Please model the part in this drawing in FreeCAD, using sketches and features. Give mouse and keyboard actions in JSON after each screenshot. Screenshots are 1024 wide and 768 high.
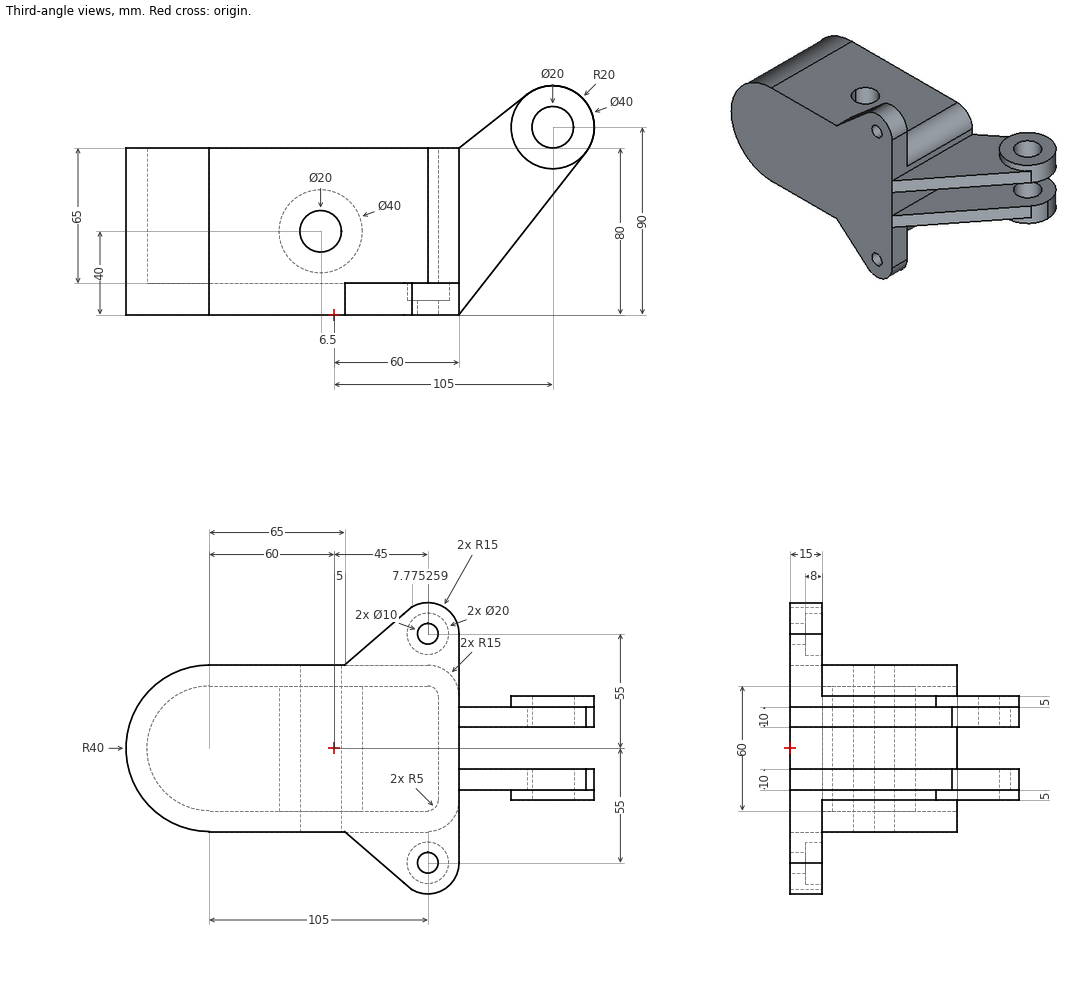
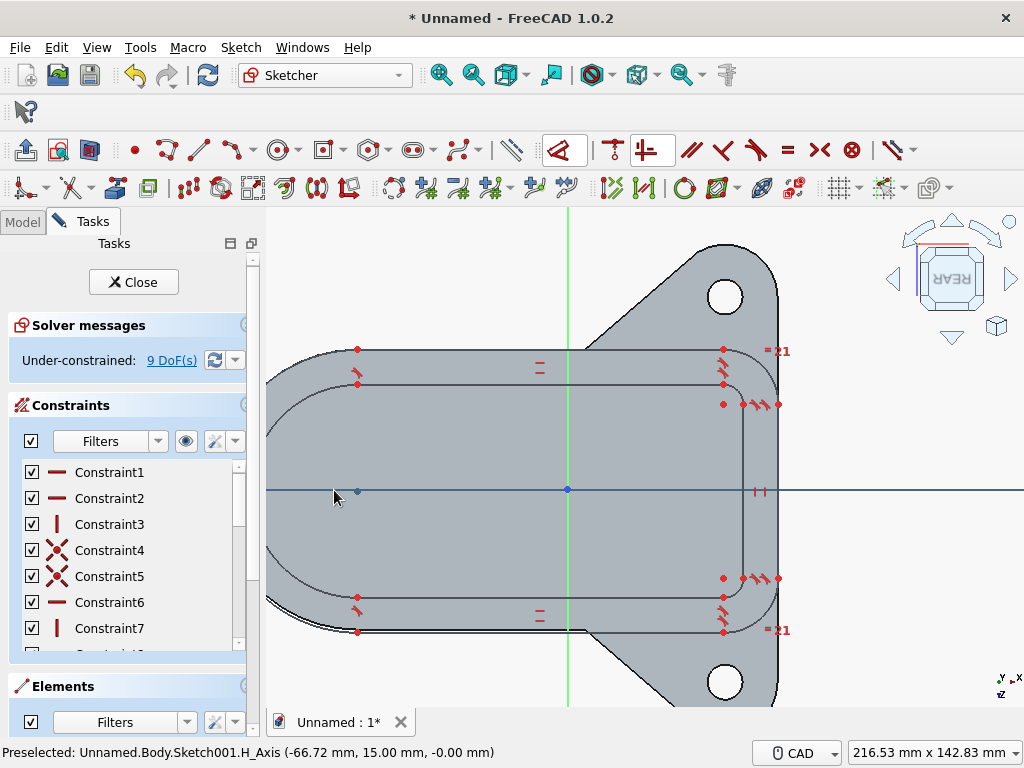
{"action": "left_click", "coordinate": [614, 150]}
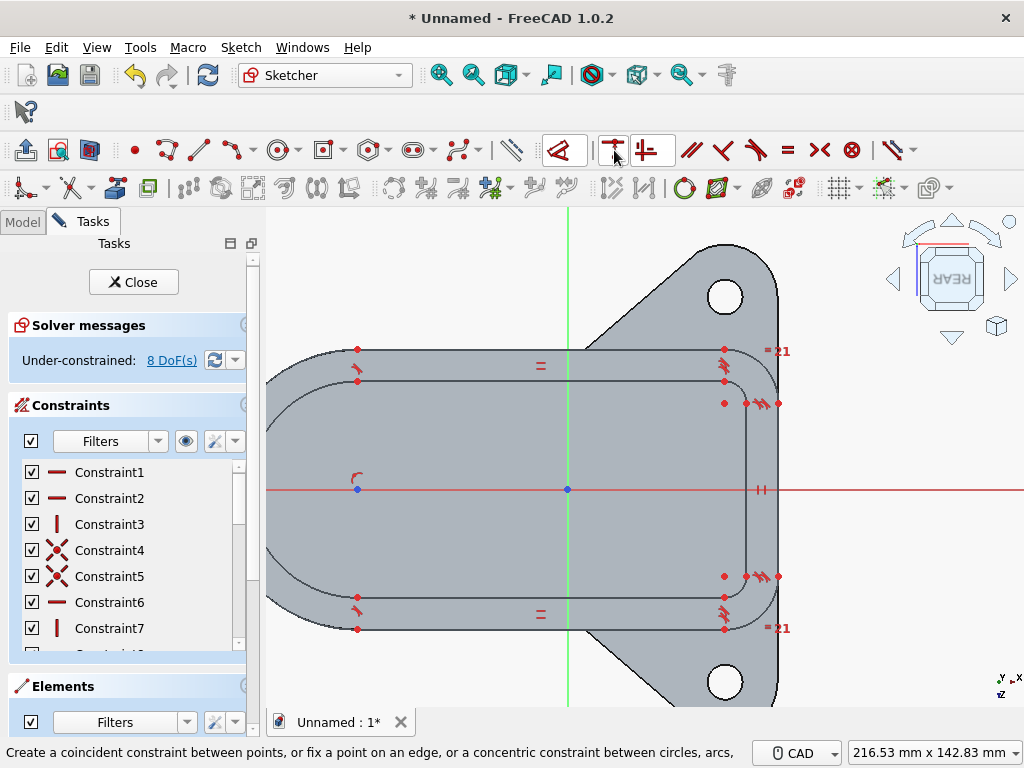
{"action": "scroll", "coordinate": [737, 391], "scroll_direction": "down", "scroll_amount": 2}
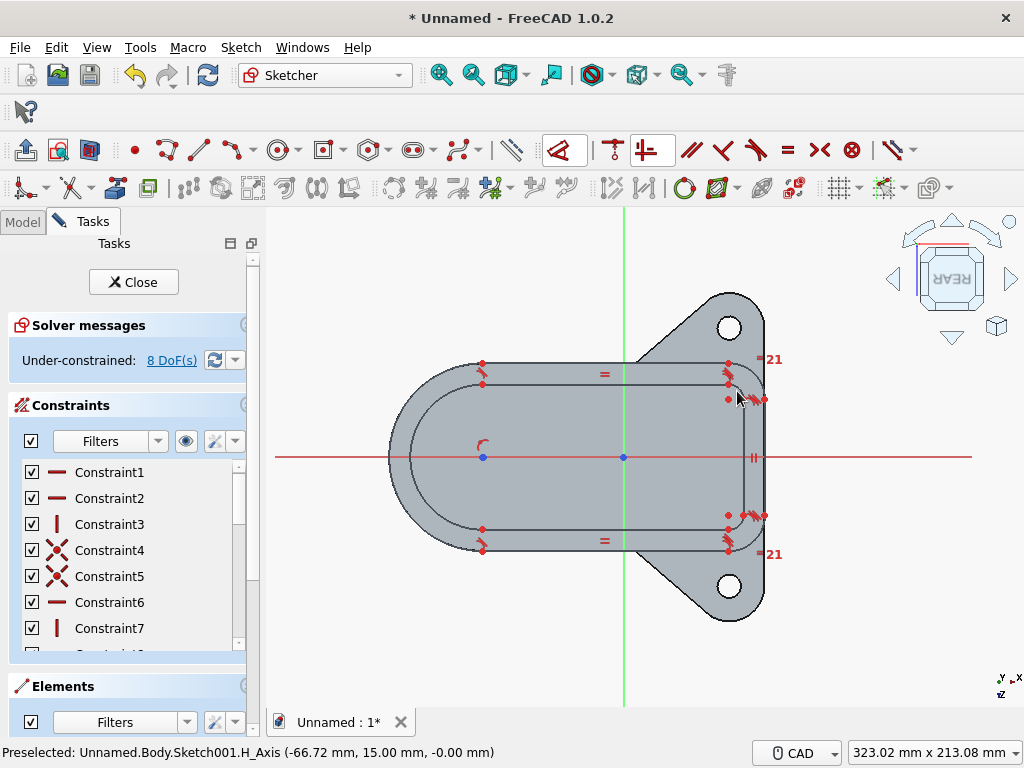
{"action": "left_click", "coordinate": [407, 402]}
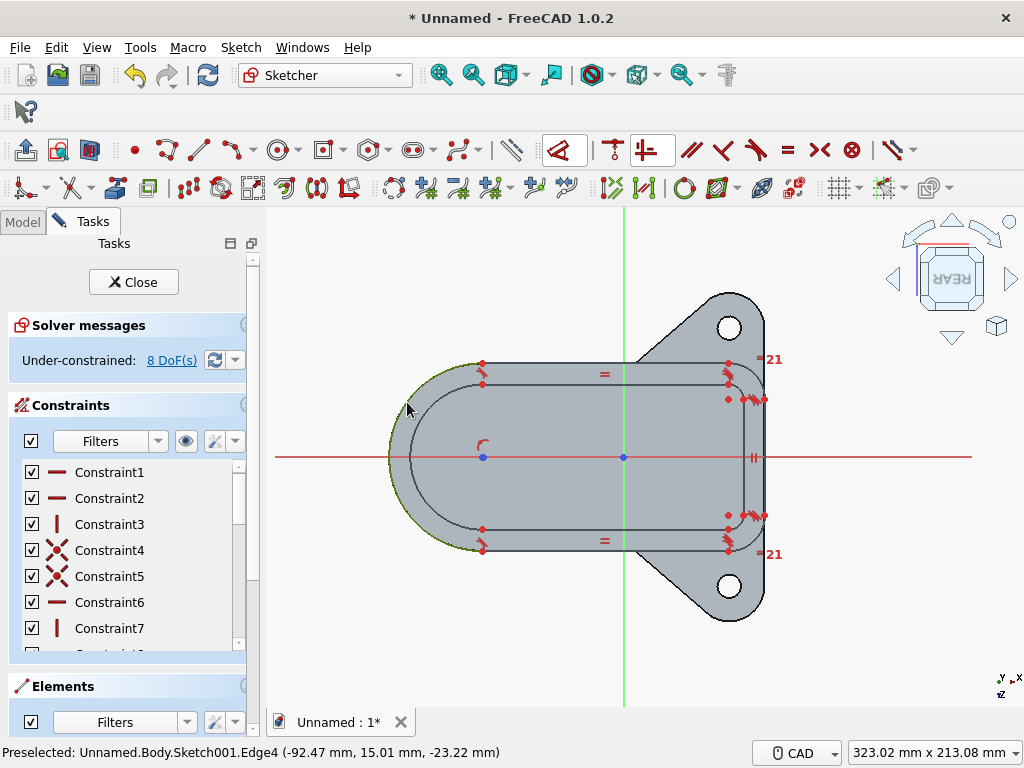
{"action": "left_click", "coordinate": [582, 150]}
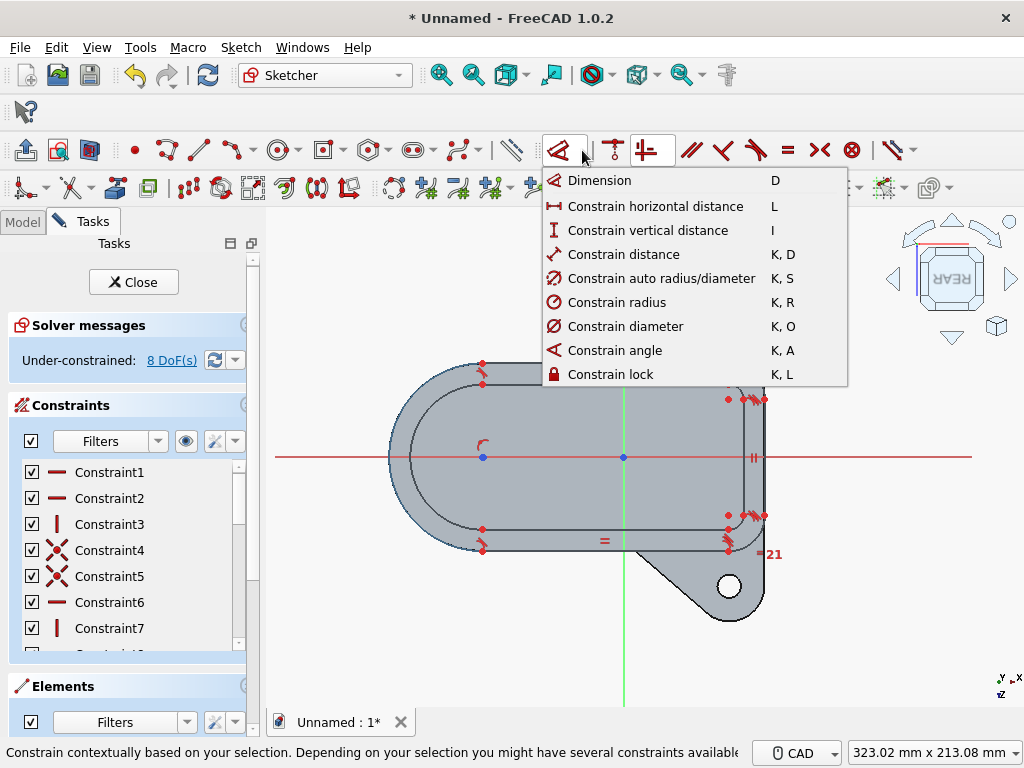
{"action": "left_click", "coordinate": [695, 302]}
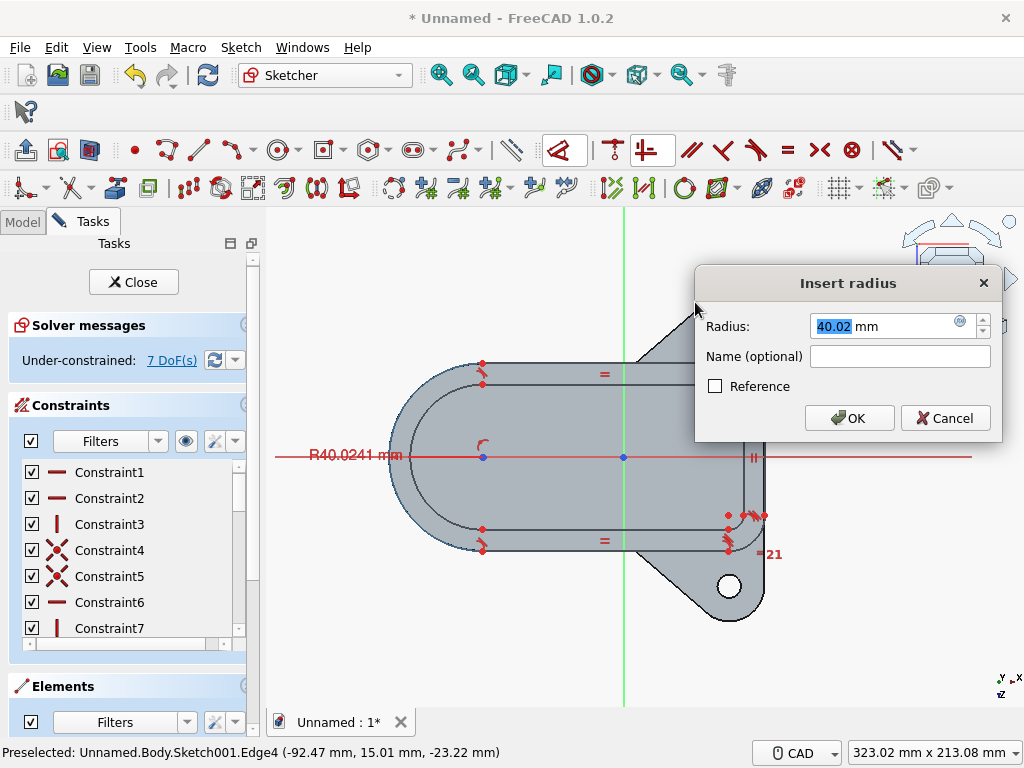
{"action": "type", "text": "40"}
{"action": "key", "text": "Return"}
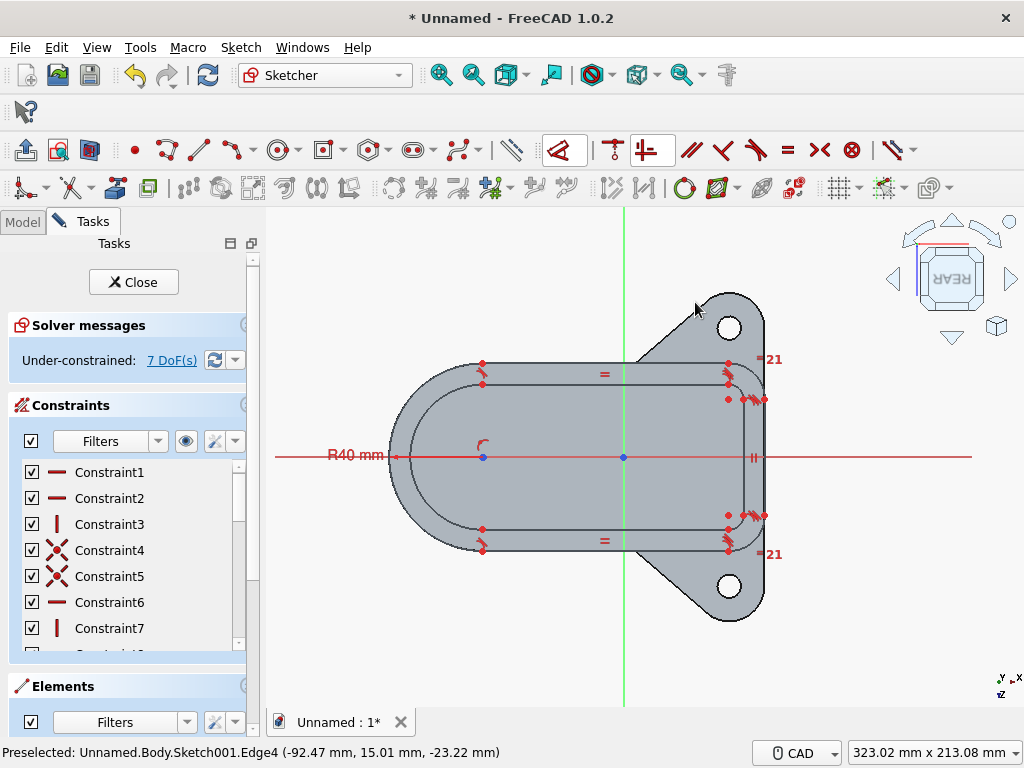
{"action": "left_click", "coordinate": [745, 547]}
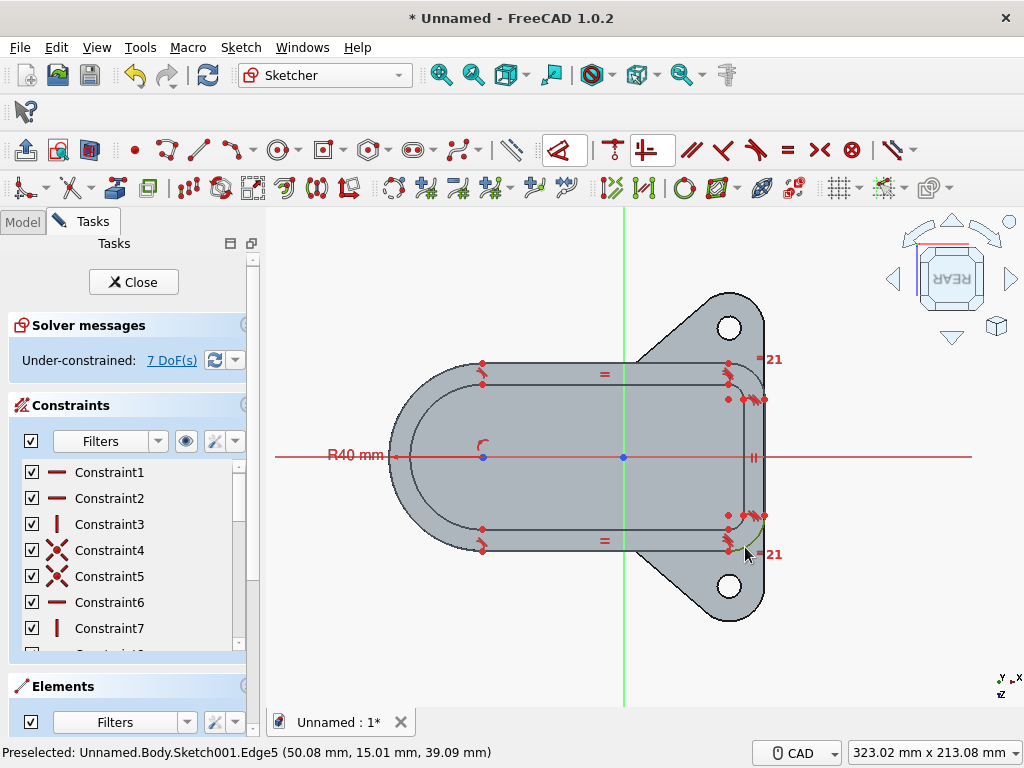
{"action": "left_click", "coordinate": [582, 150]}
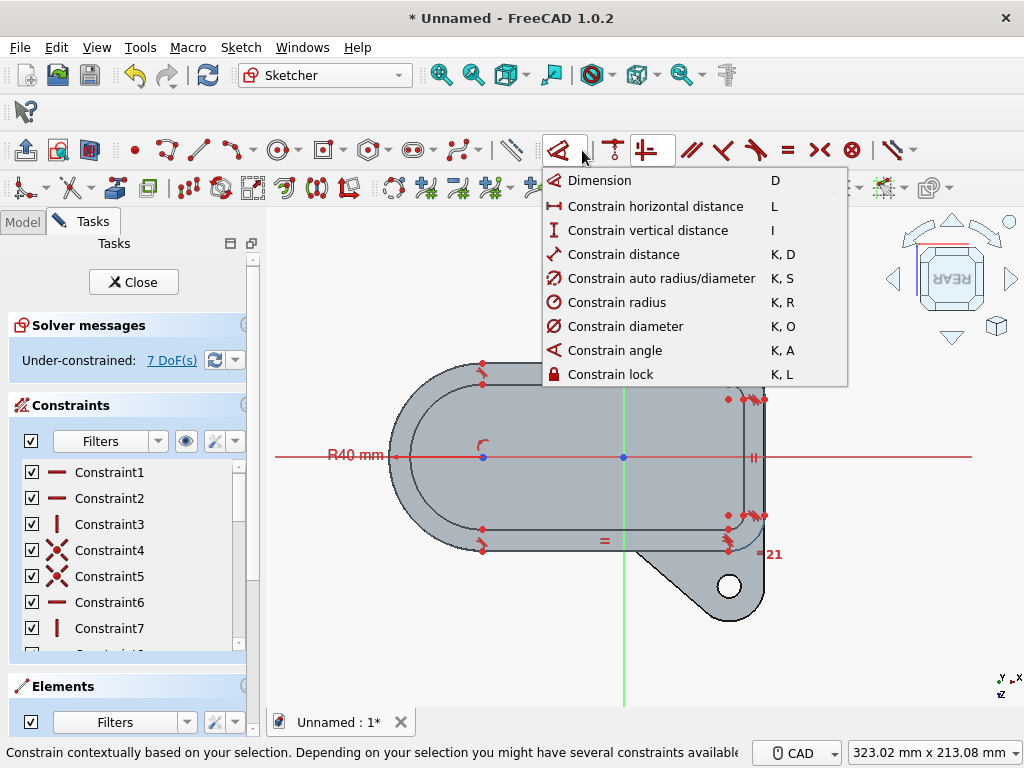
{"action": "left_click", "coordinate": [695, 302]}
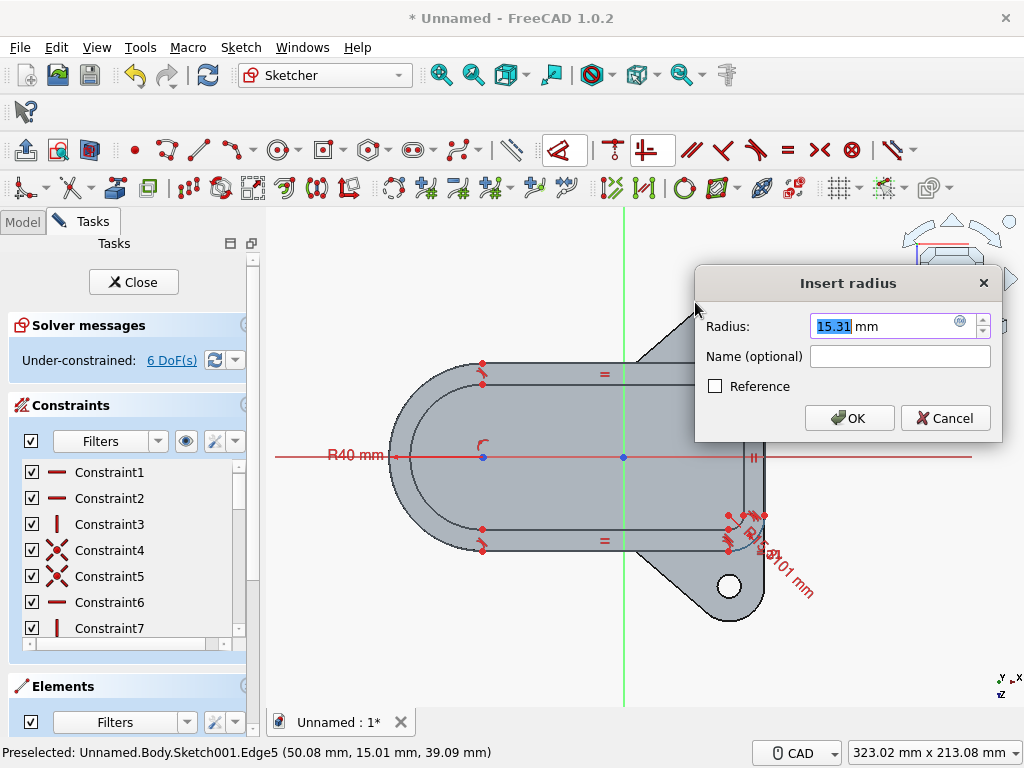
{"action": "type", "text": "15"}
{"action": "key", "text": "Return"}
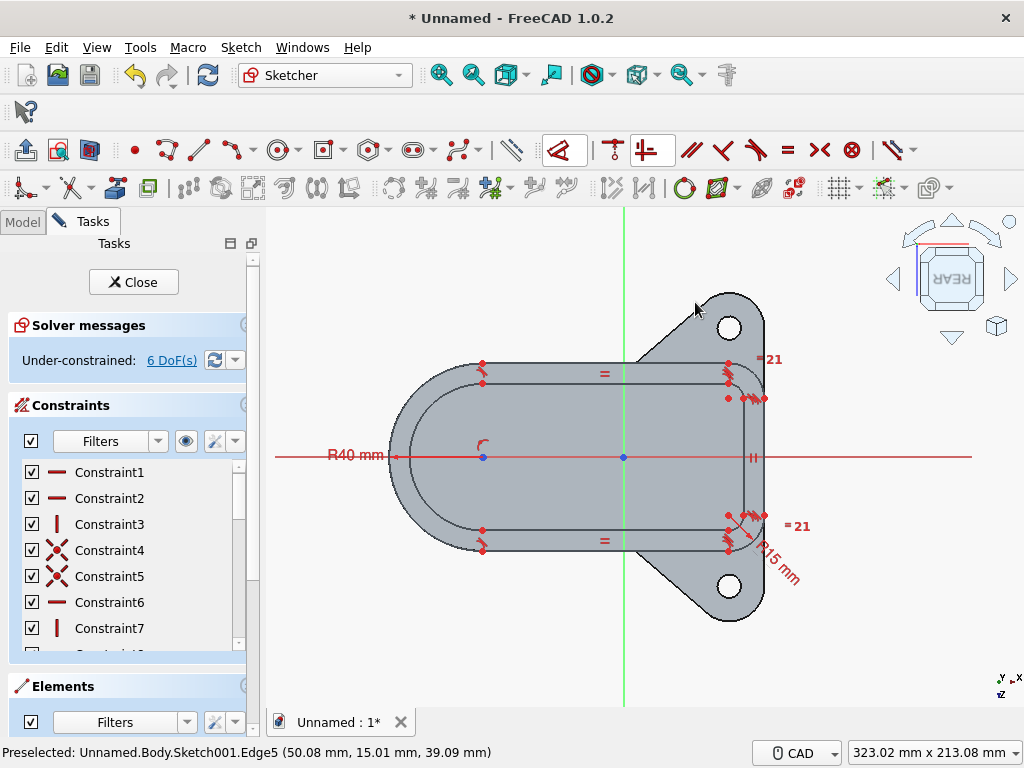
{"action": "scroll", "coordinate": [739, 388], "scroll_direction": "up", "scroll_amount": 7}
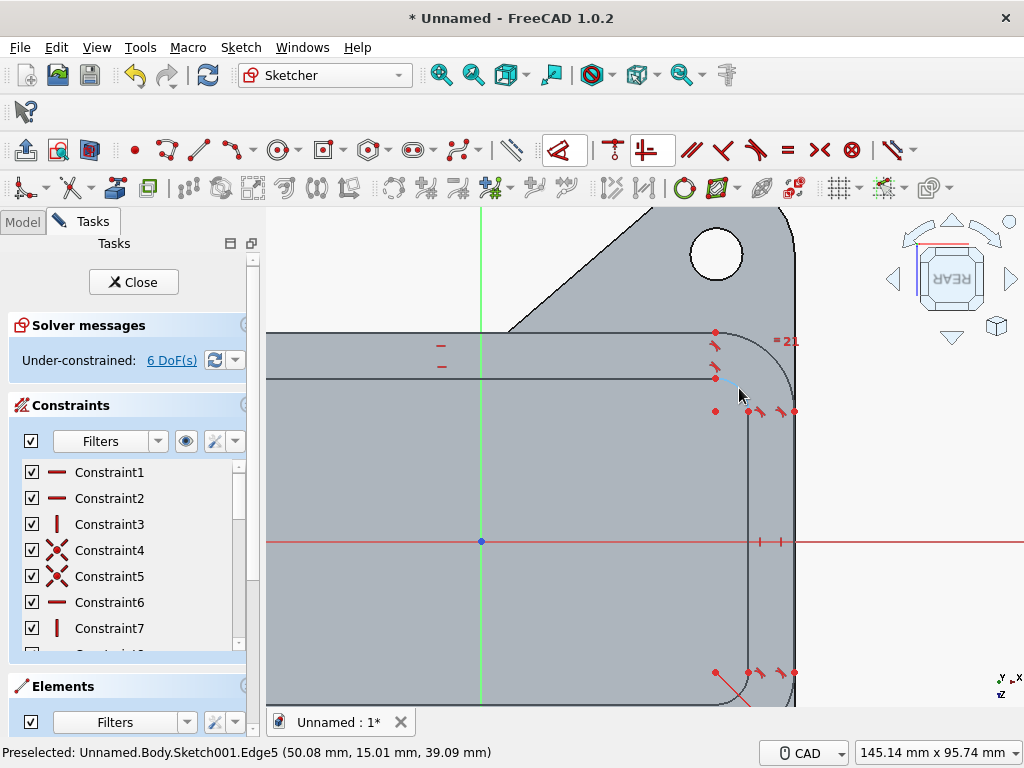
{"action": "left_click", "coordinate": [738, 388]}